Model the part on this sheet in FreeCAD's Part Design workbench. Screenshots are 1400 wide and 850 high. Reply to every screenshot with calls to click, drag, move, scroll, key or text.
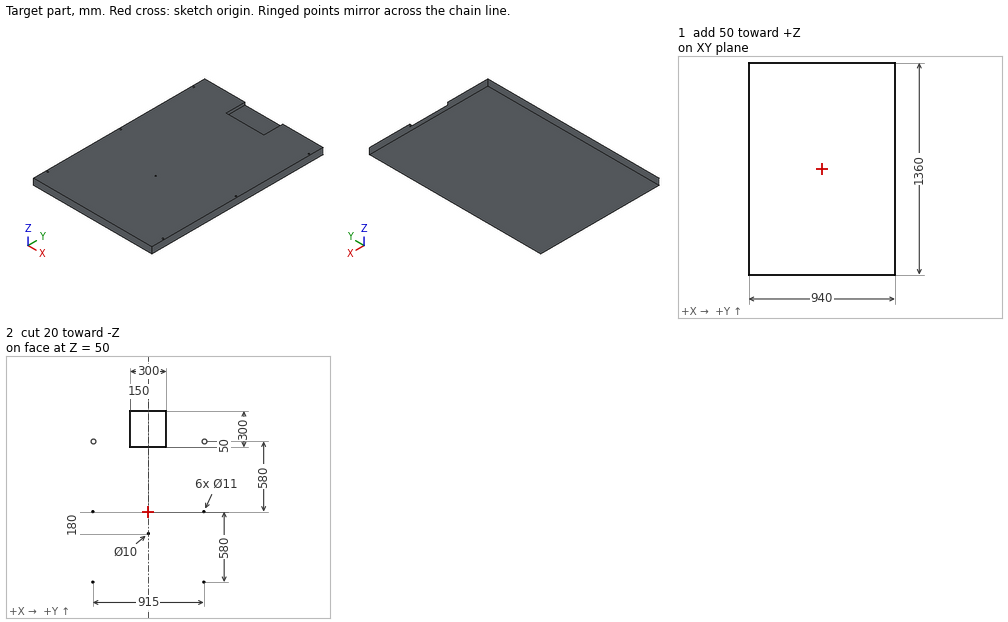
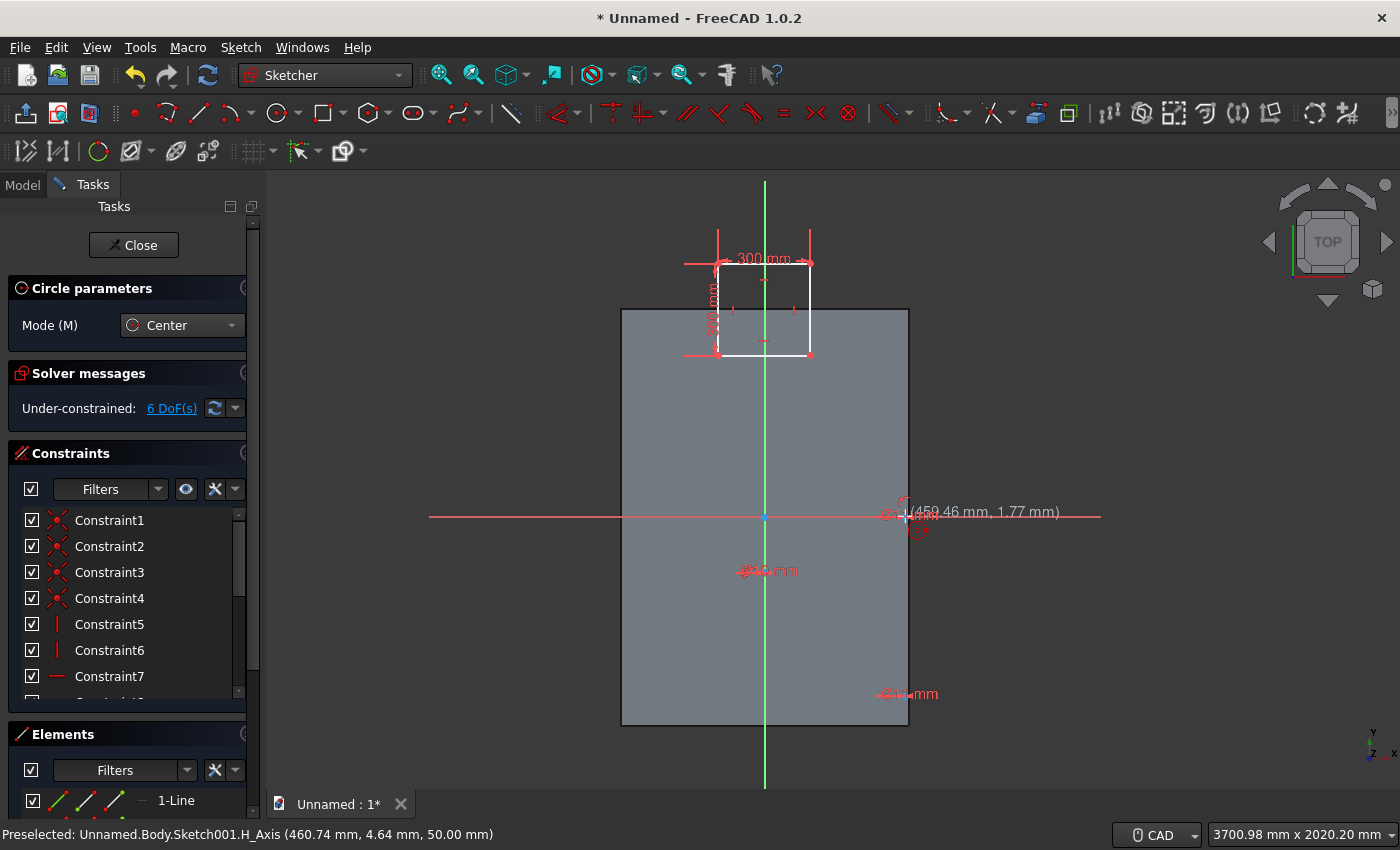
scroll(905, 339, up, 13)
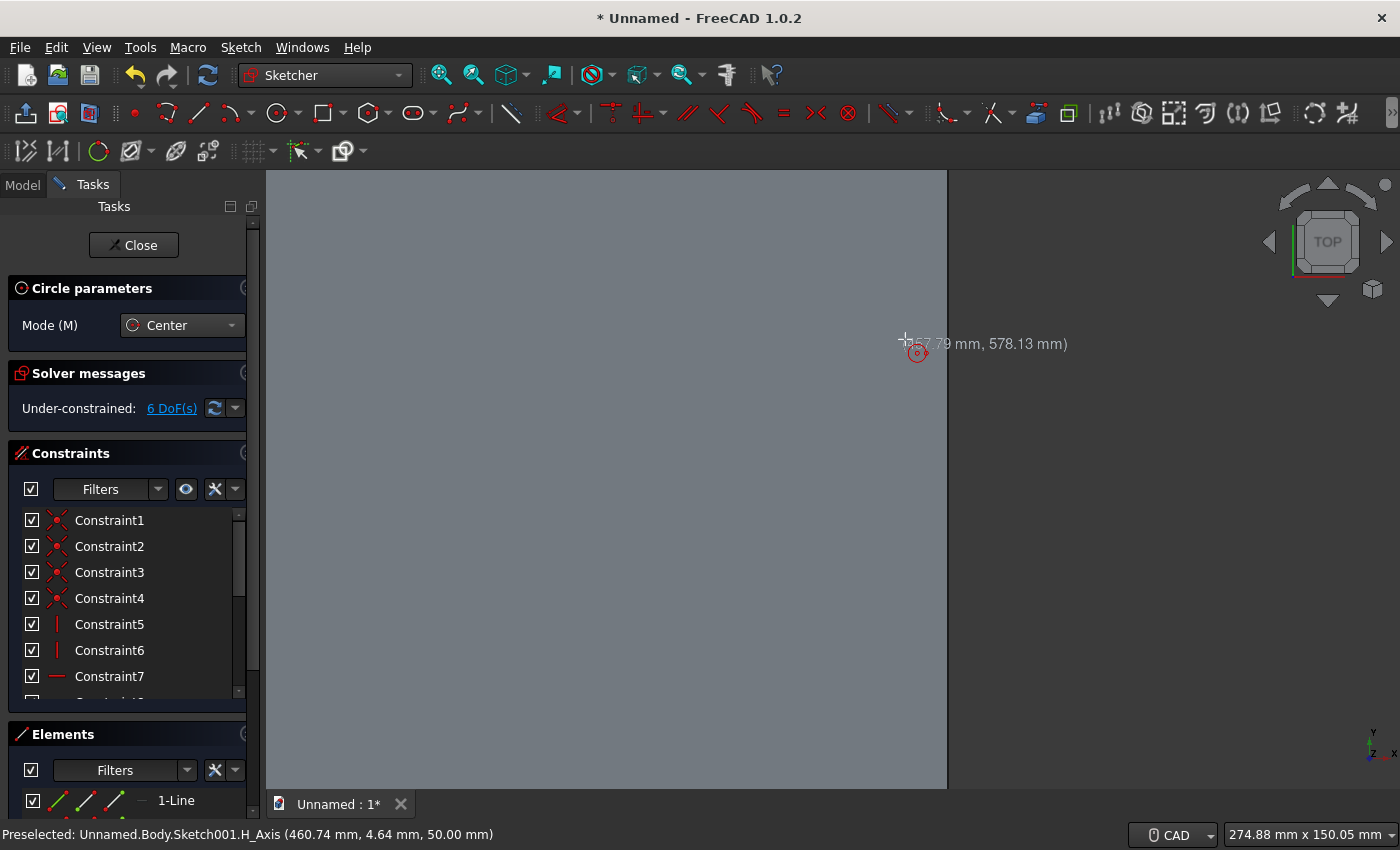
scroll(905, 339, down, 13)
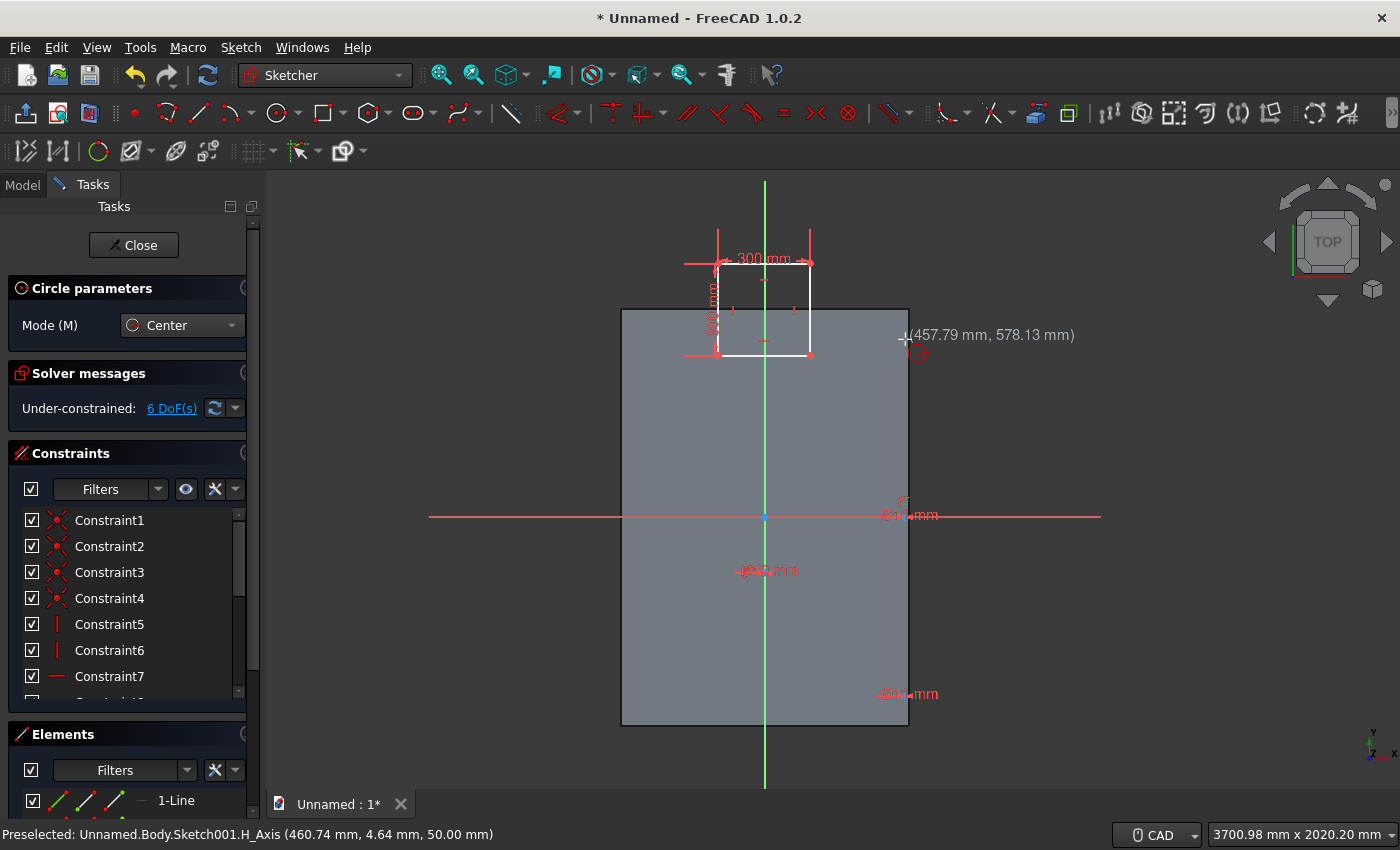
click(905, 339)
move(906, 338)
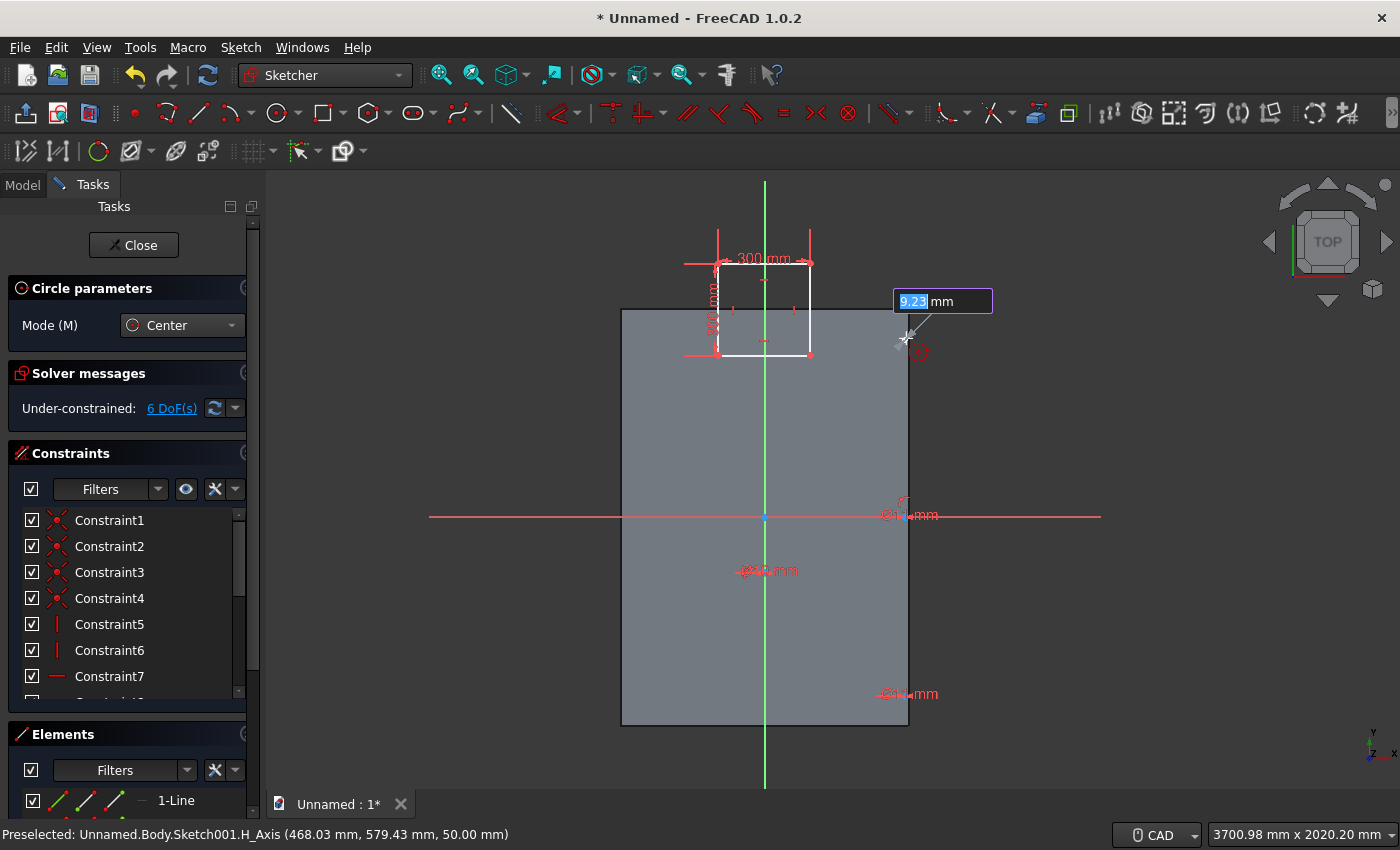
text(11)
key(Return)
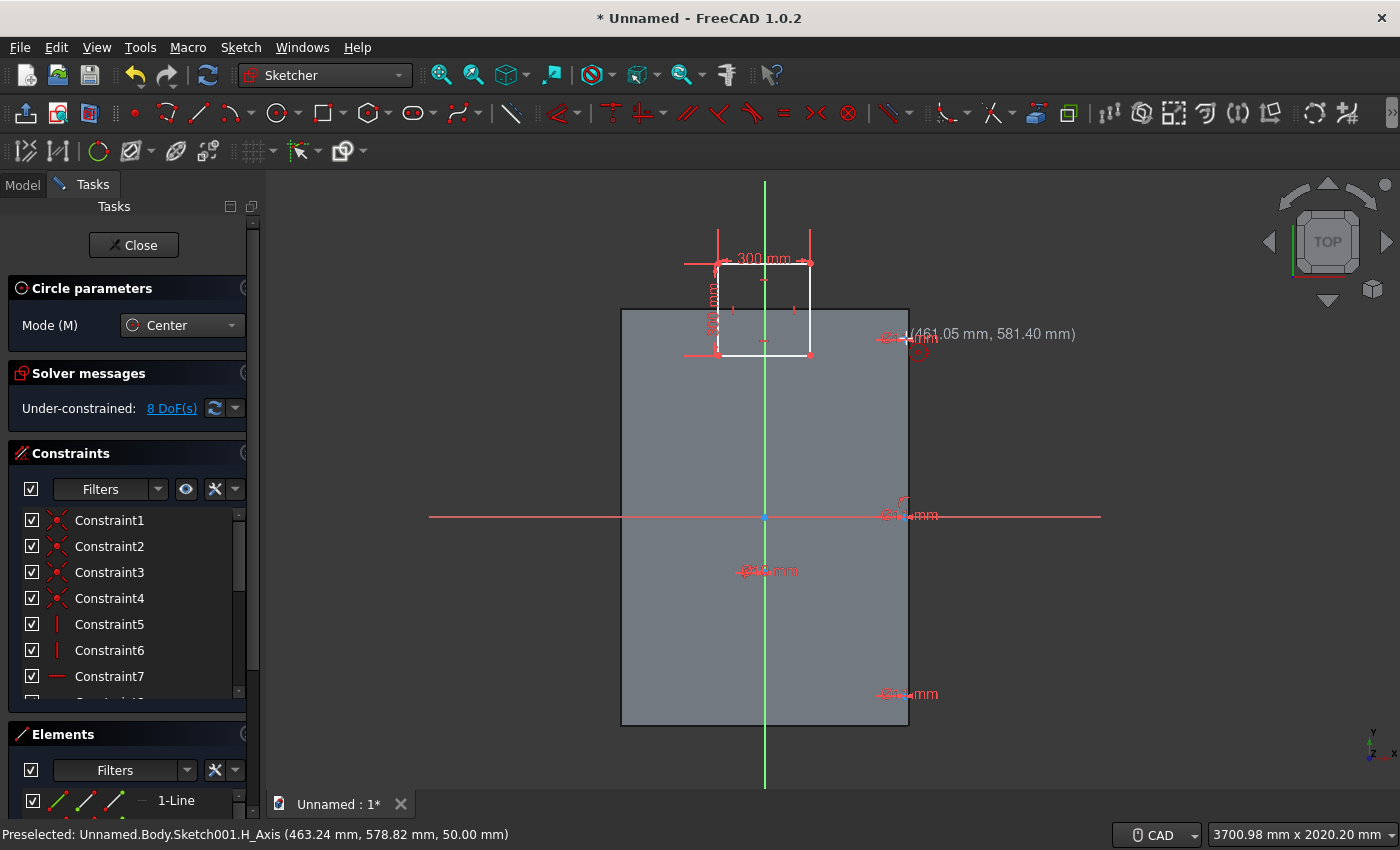
scroll(625, 339, up, 13)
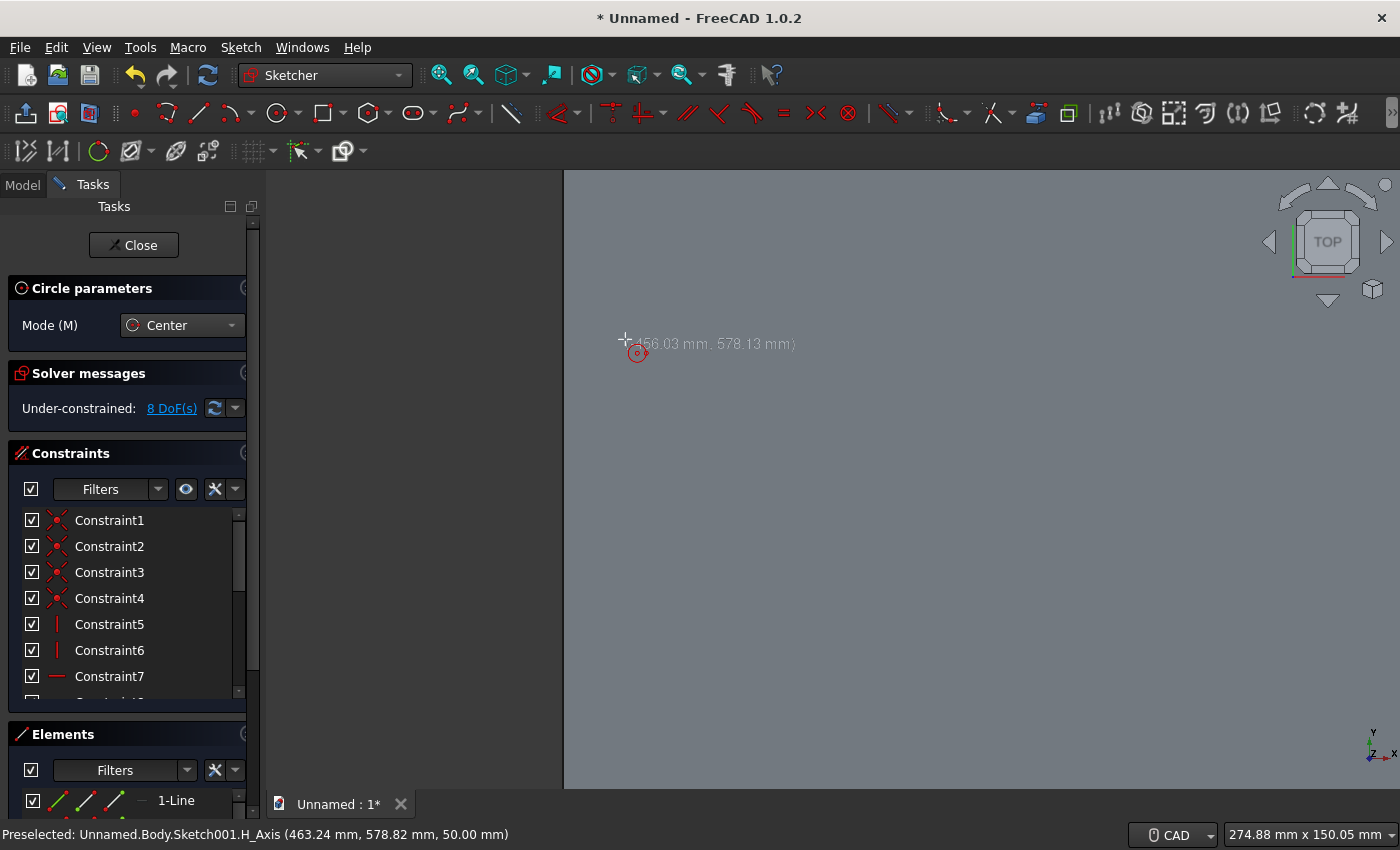
scroll(625, 339, down, 13)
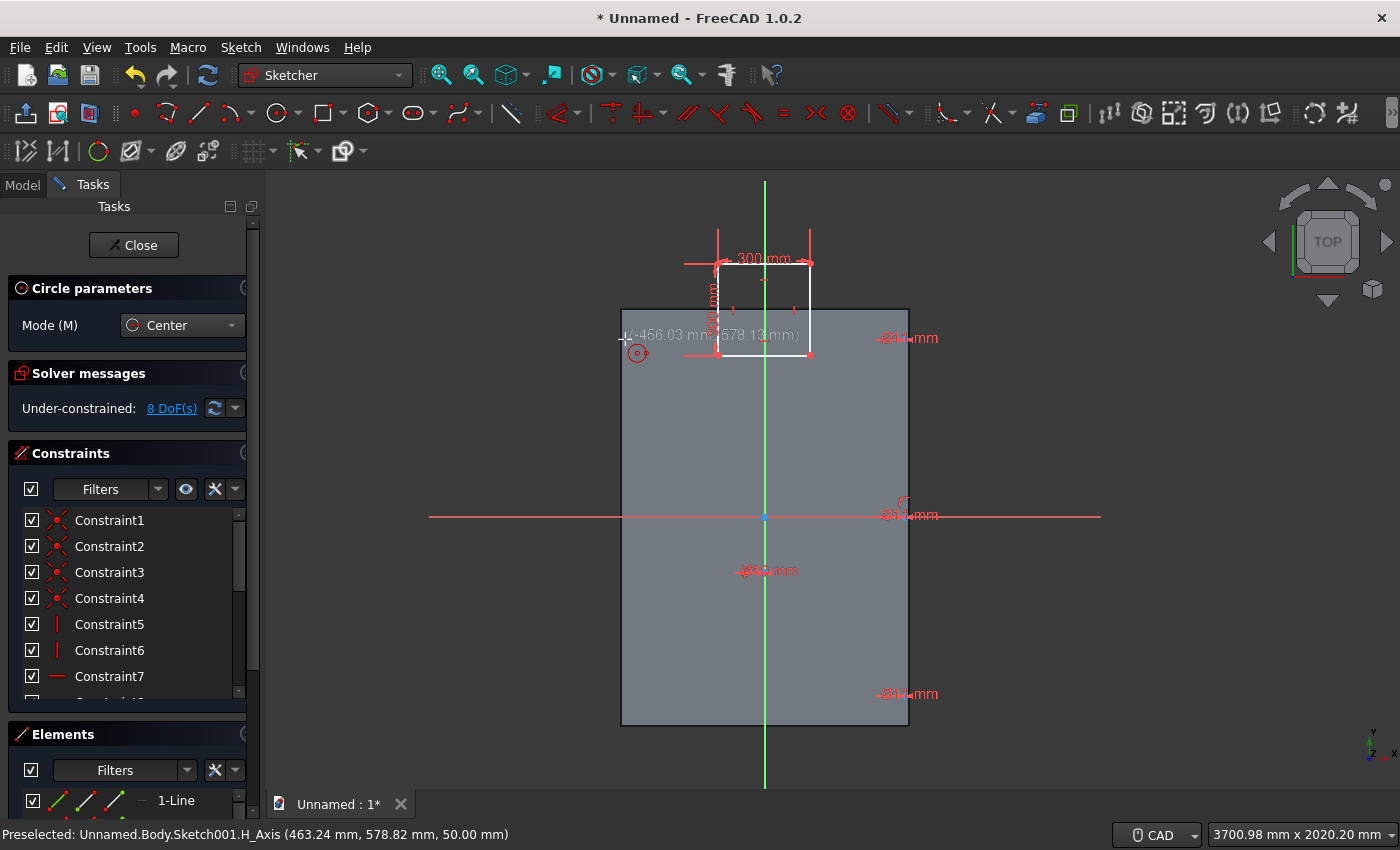
click(625, 339)
move(626, 338)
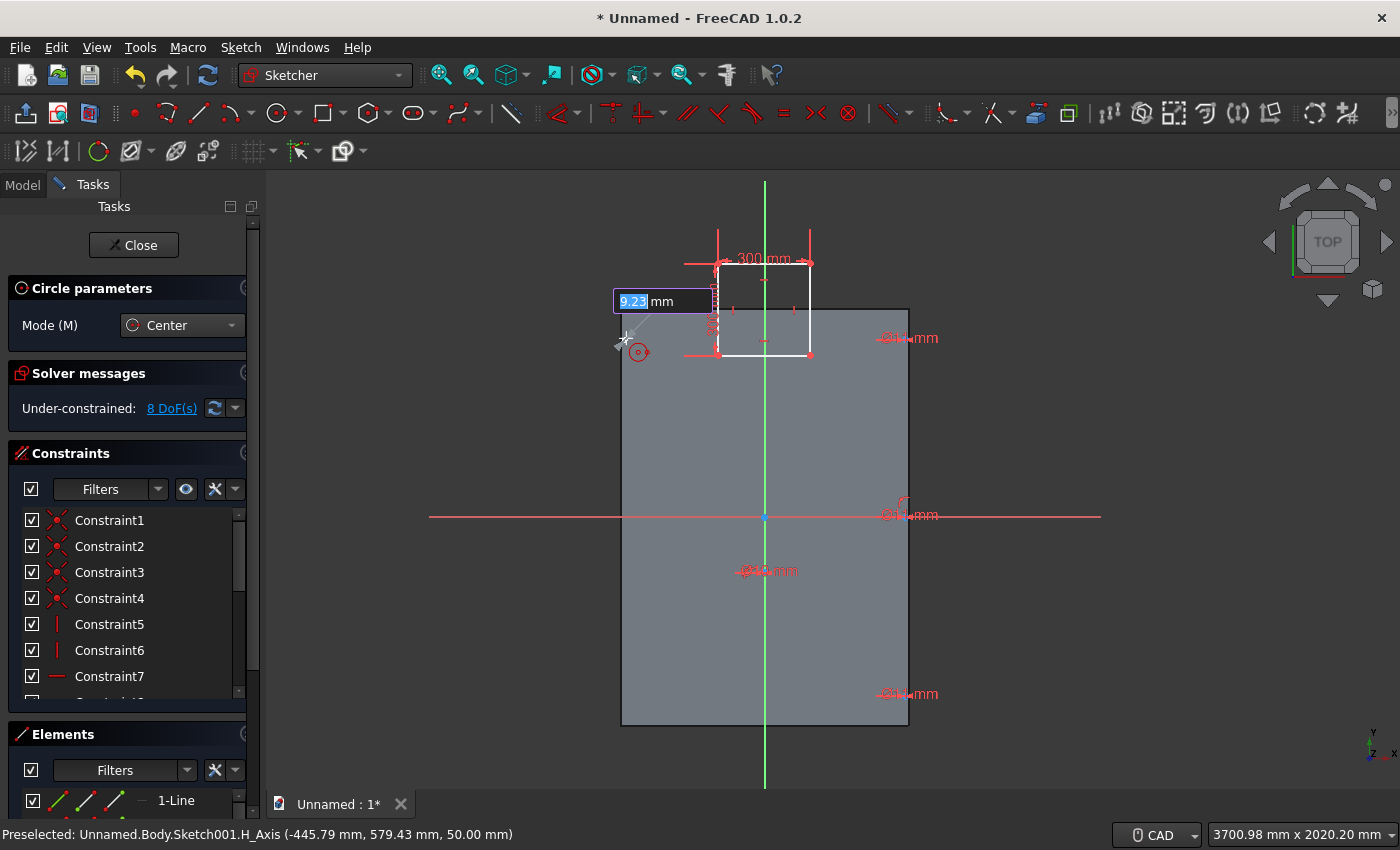
text(11)
key(Return)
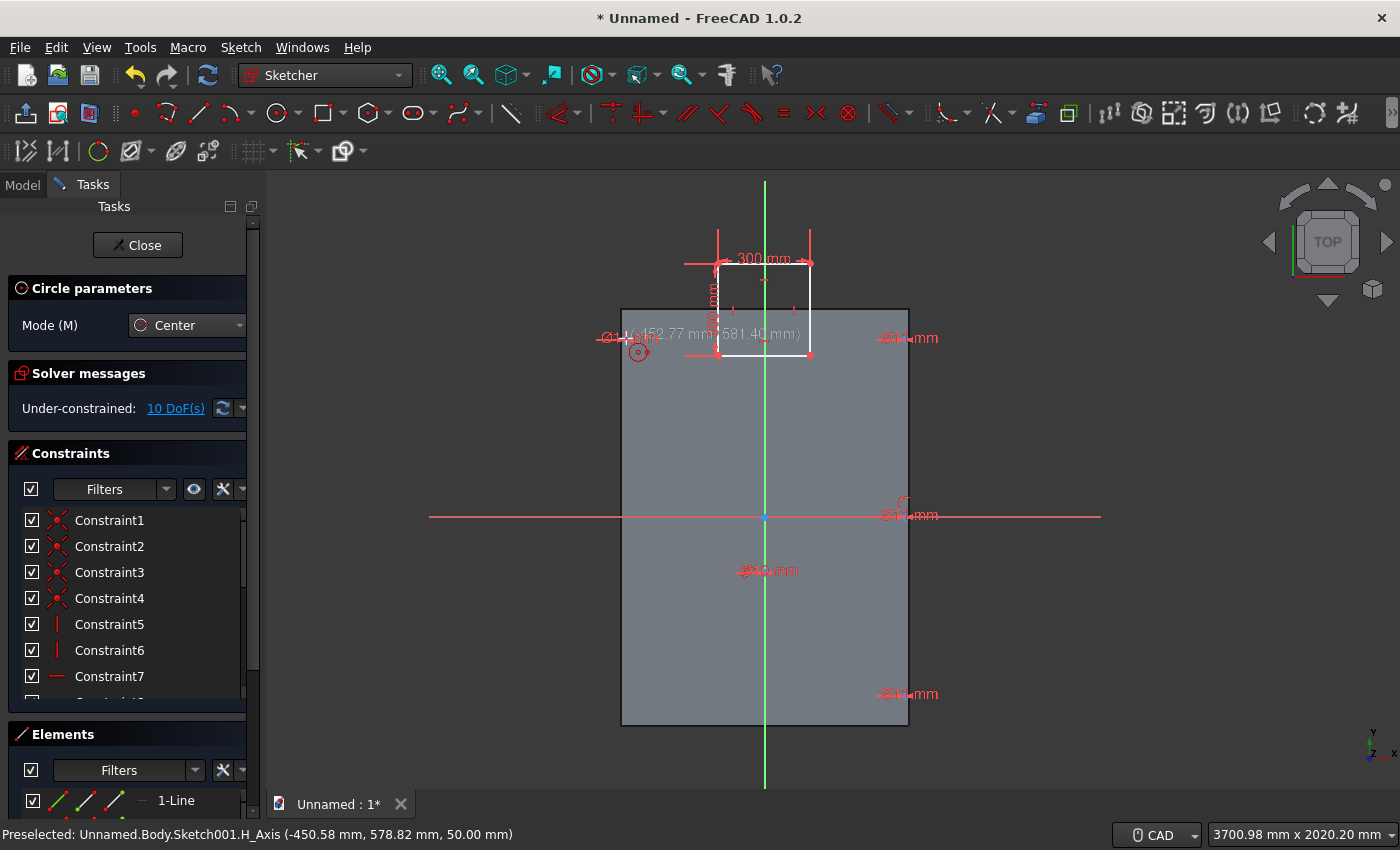
scroll(625, 517, up, 13)